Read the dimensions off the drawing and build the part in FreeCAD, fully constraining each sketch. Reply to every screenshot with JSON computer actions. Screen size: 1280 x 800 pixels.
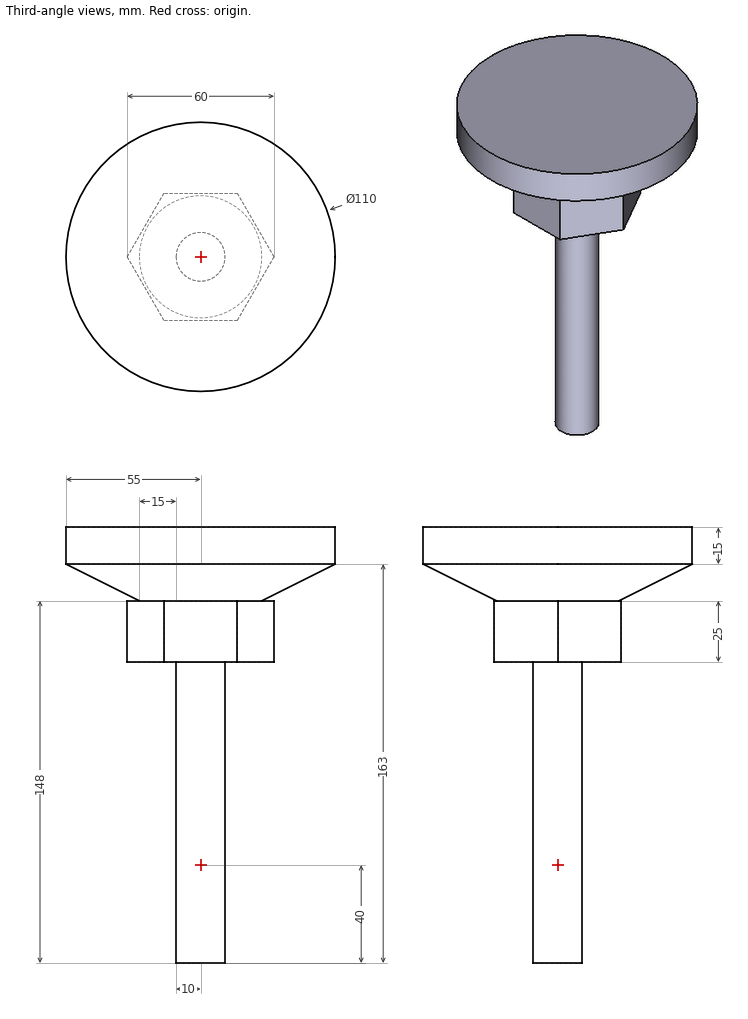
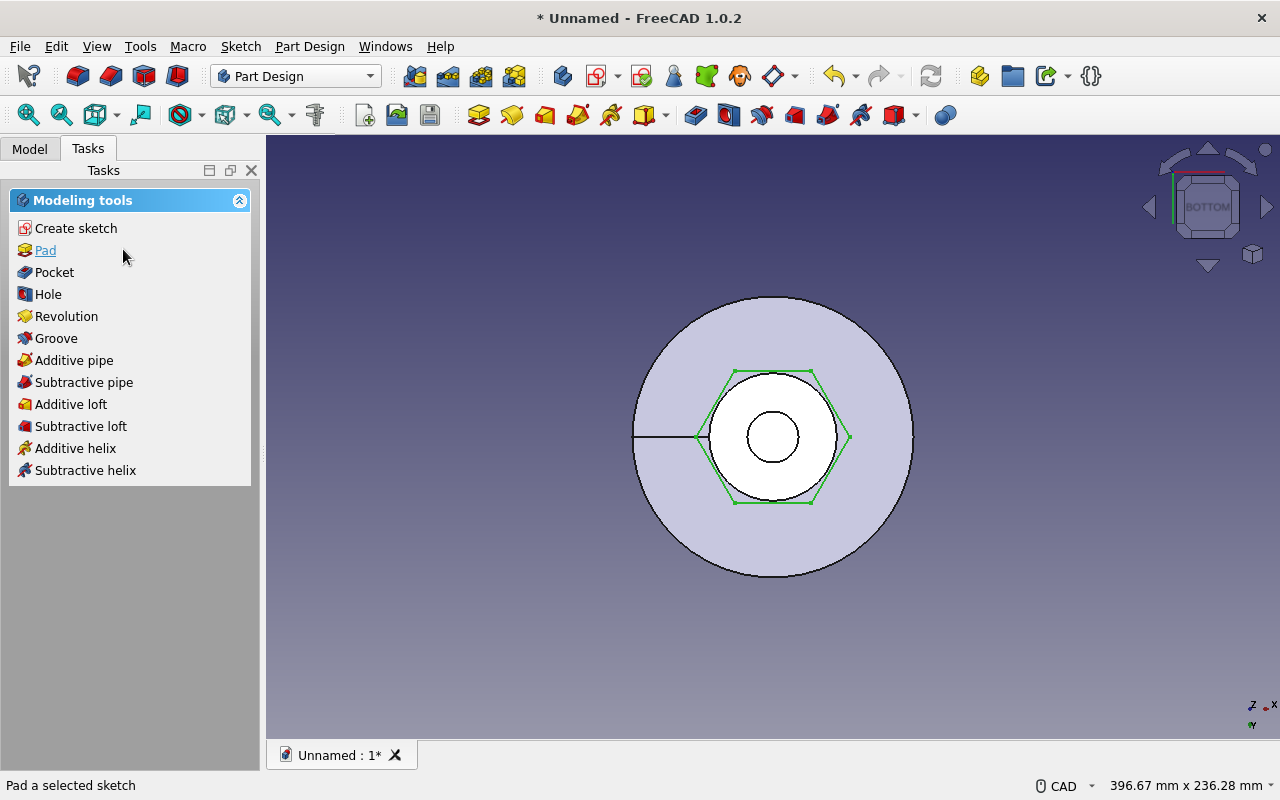
{"action": "left_click", "coordinate": [479, 116]}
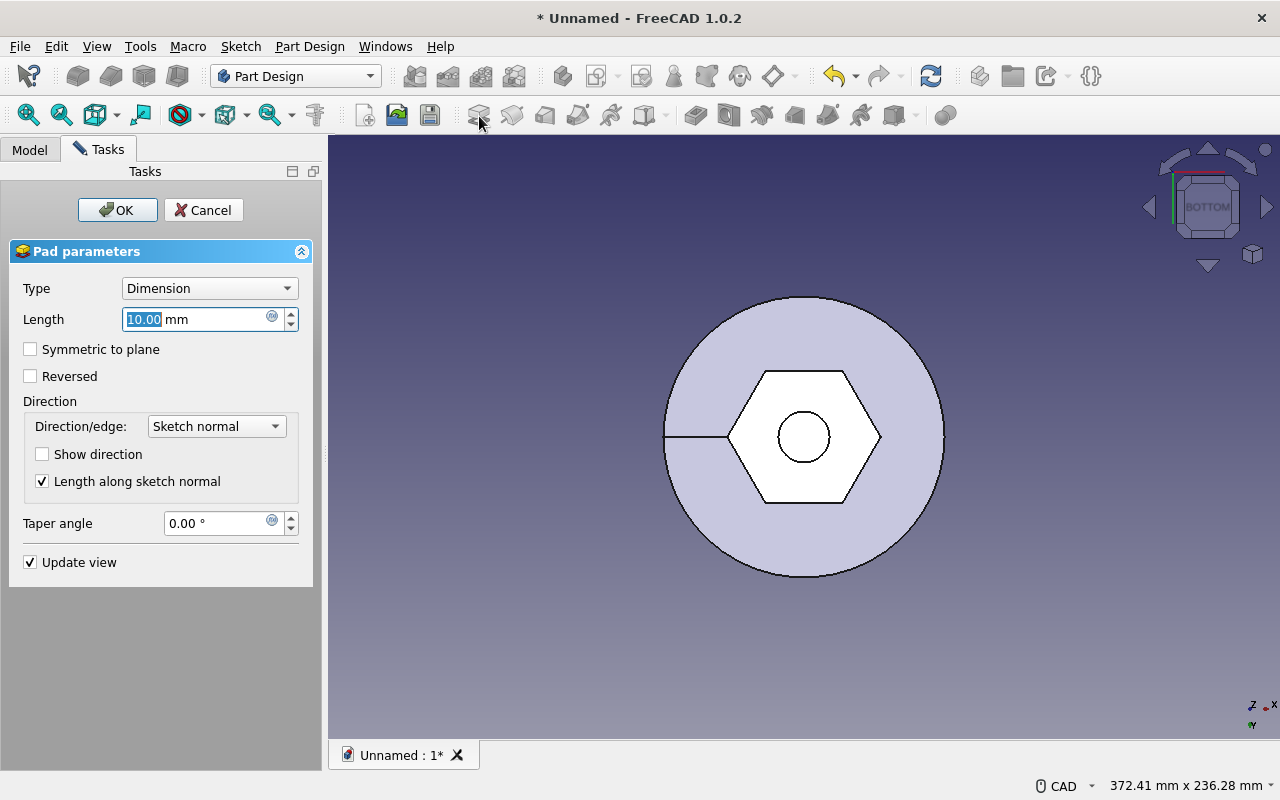
{"action": "type", "text": "25"}
{"action": "key", "text": "Tab"}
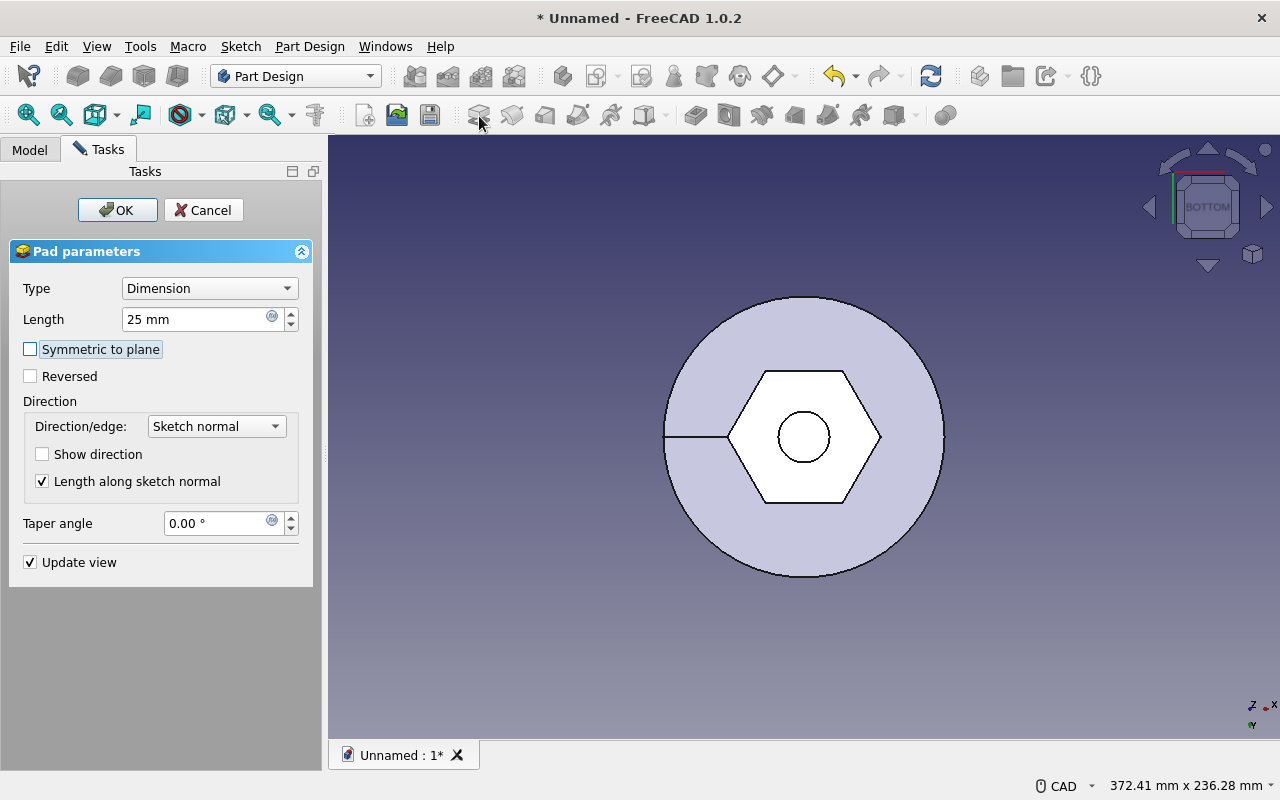
{"action": "left_click", "coordinate": [118, 210]}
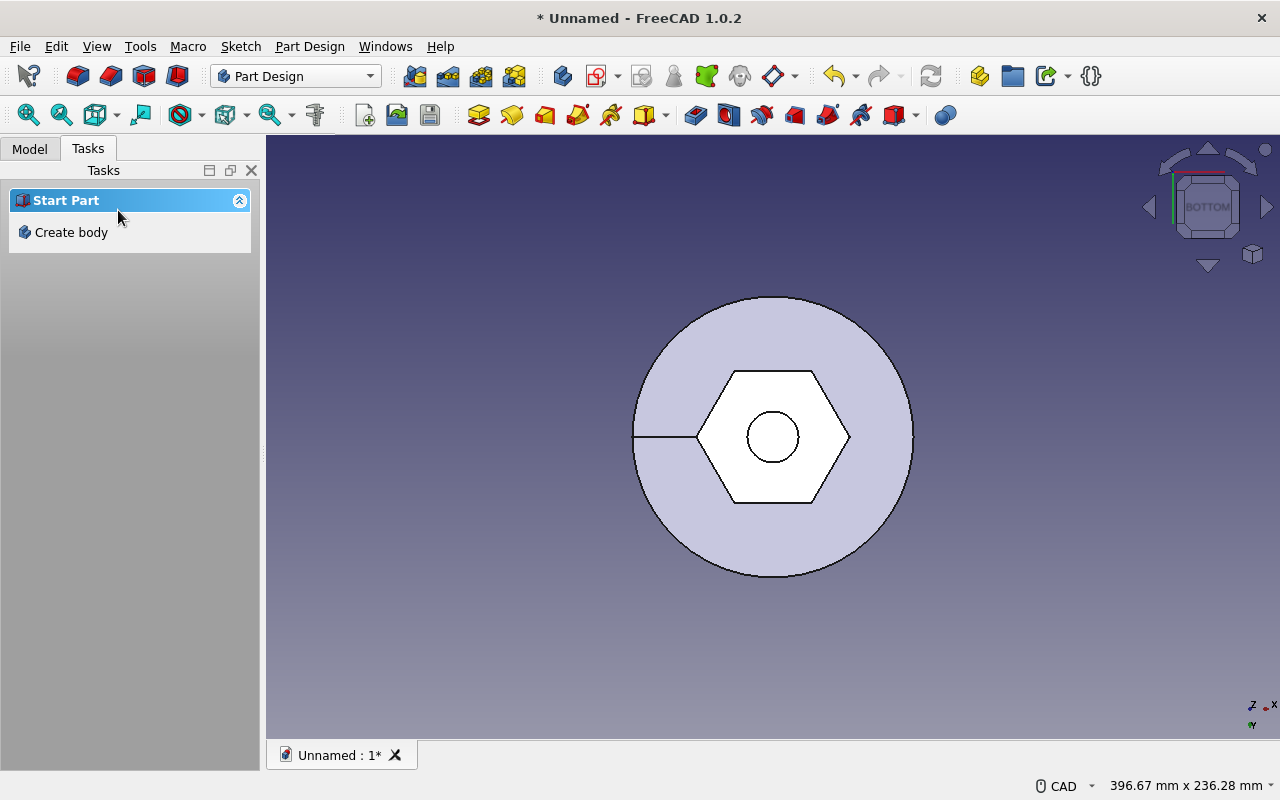
{"action": "key", "text": "0"}